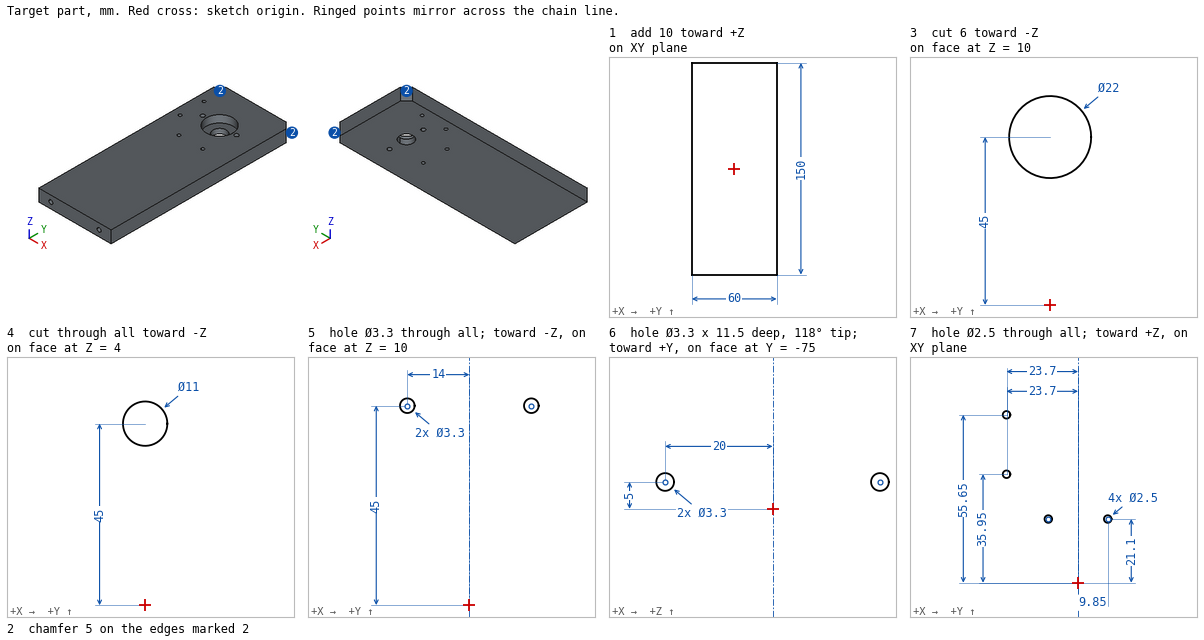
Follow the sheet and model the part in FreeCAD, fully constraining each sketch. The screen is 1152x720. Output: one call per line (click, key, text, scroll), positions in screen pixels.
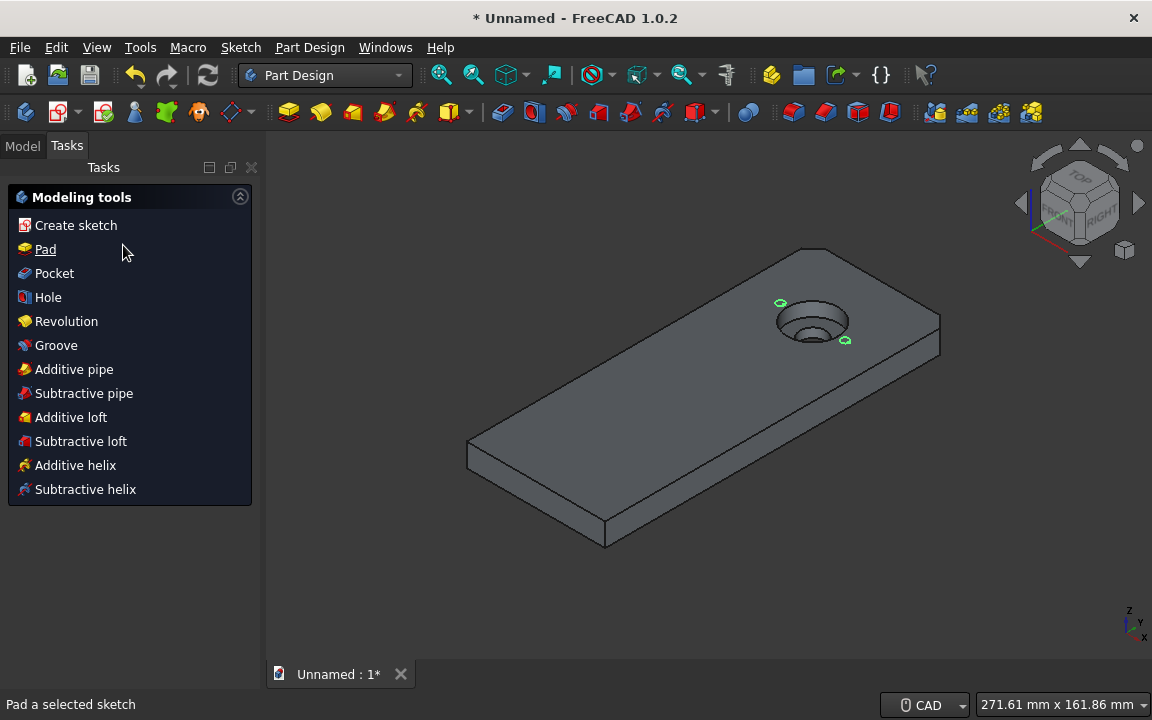
click(536, 112)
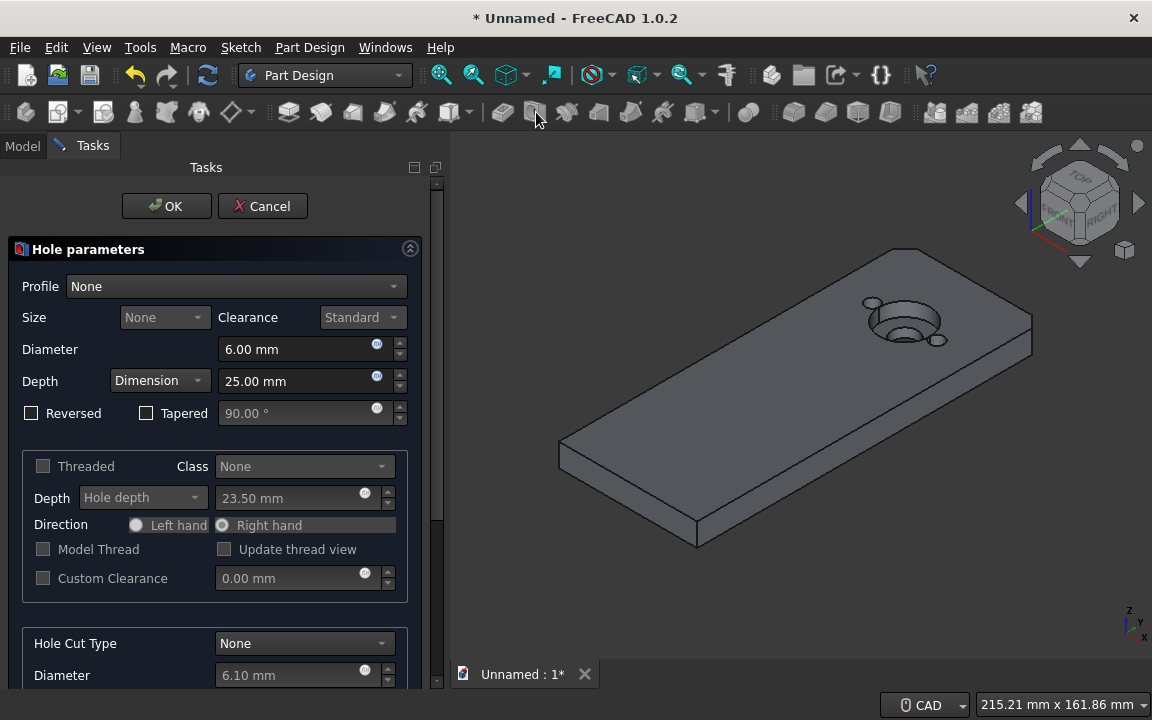
triple_click(305, 349)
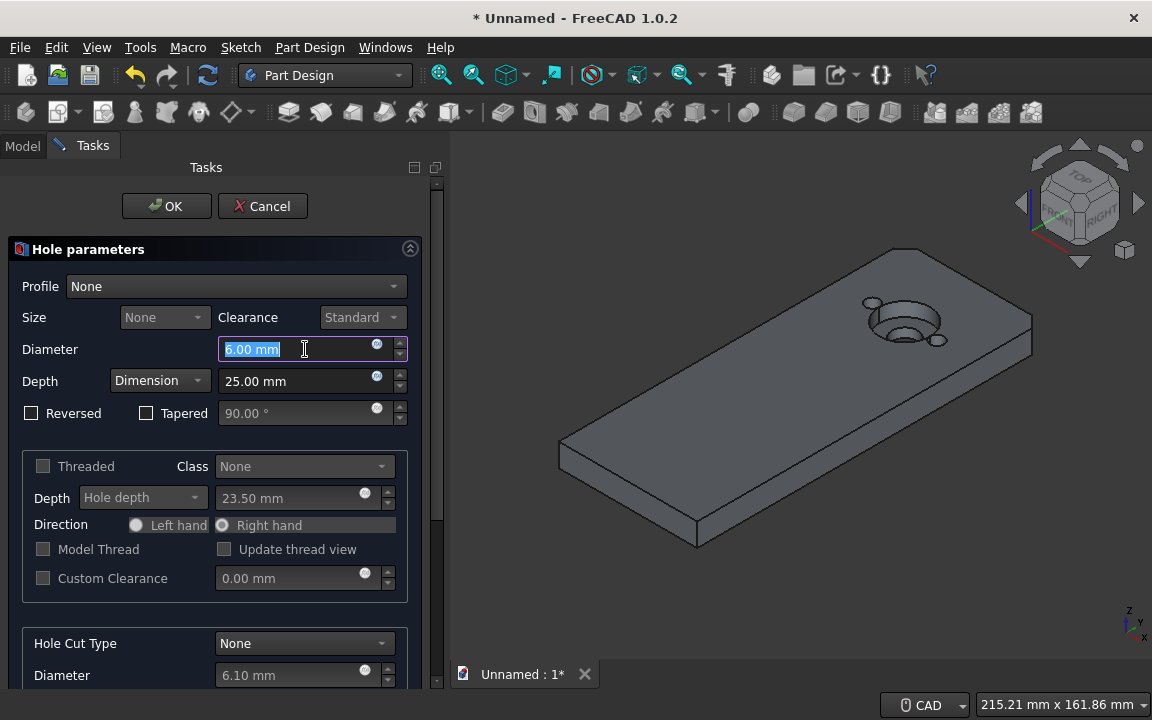
text(3.3)
key(Tab)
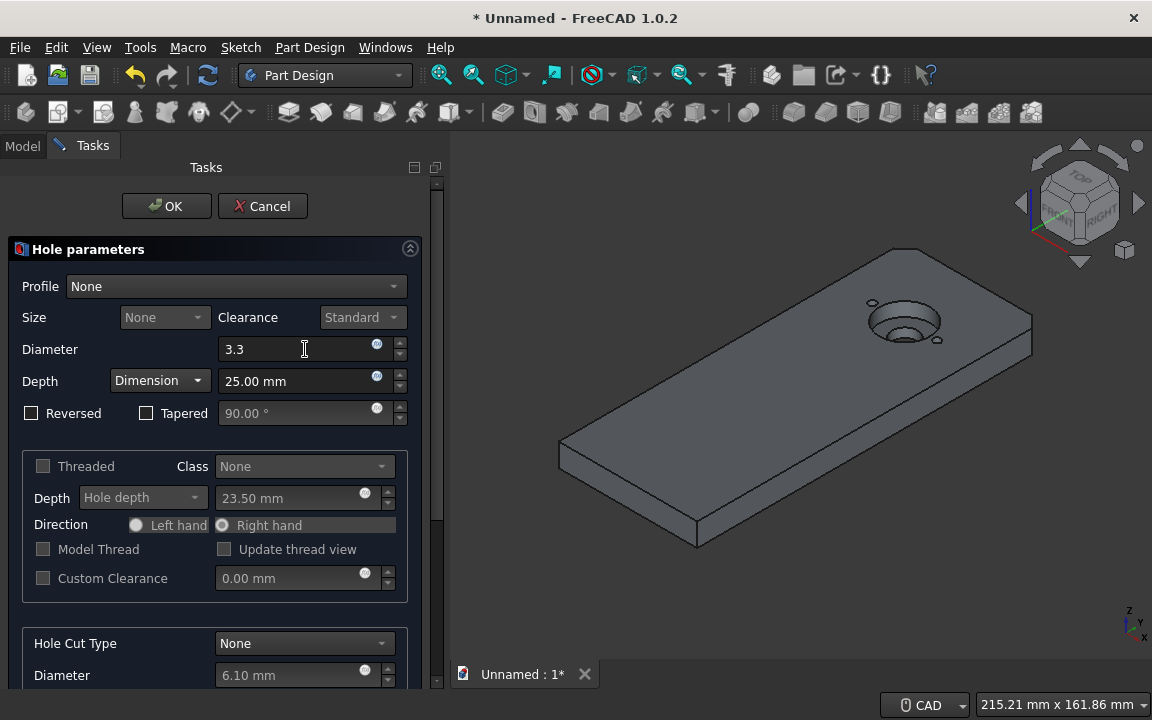
click(161, 380)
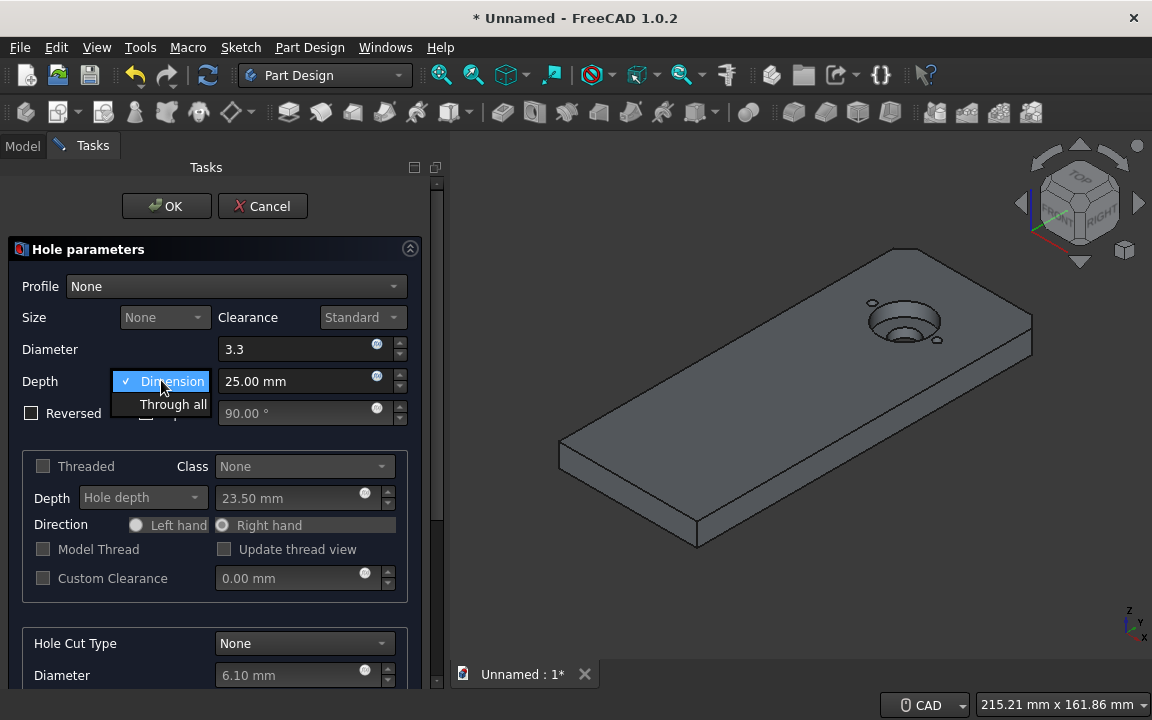
click(160, 404)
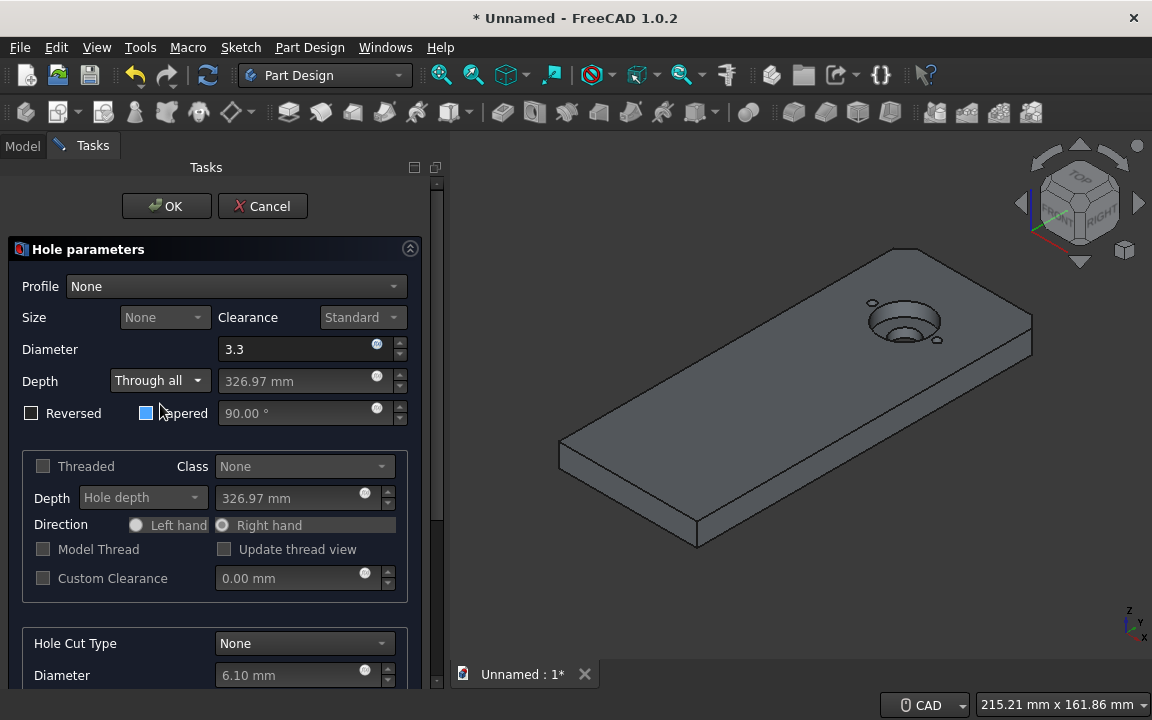
click(167, 206)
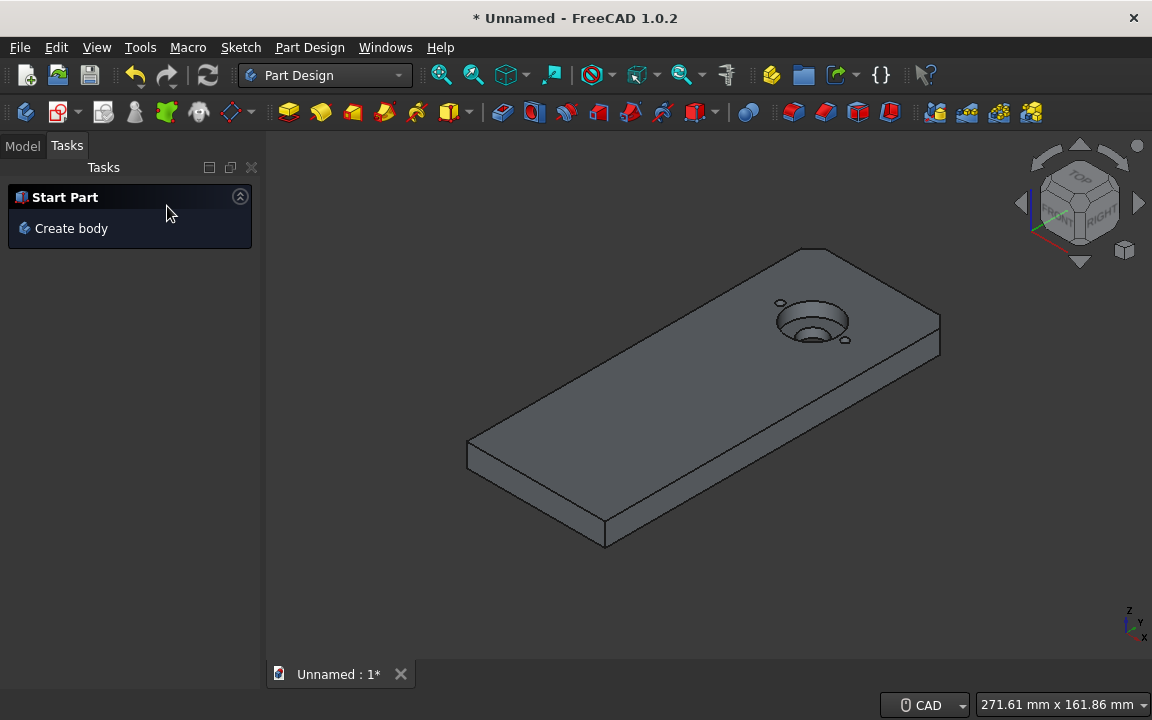
click(576, 517)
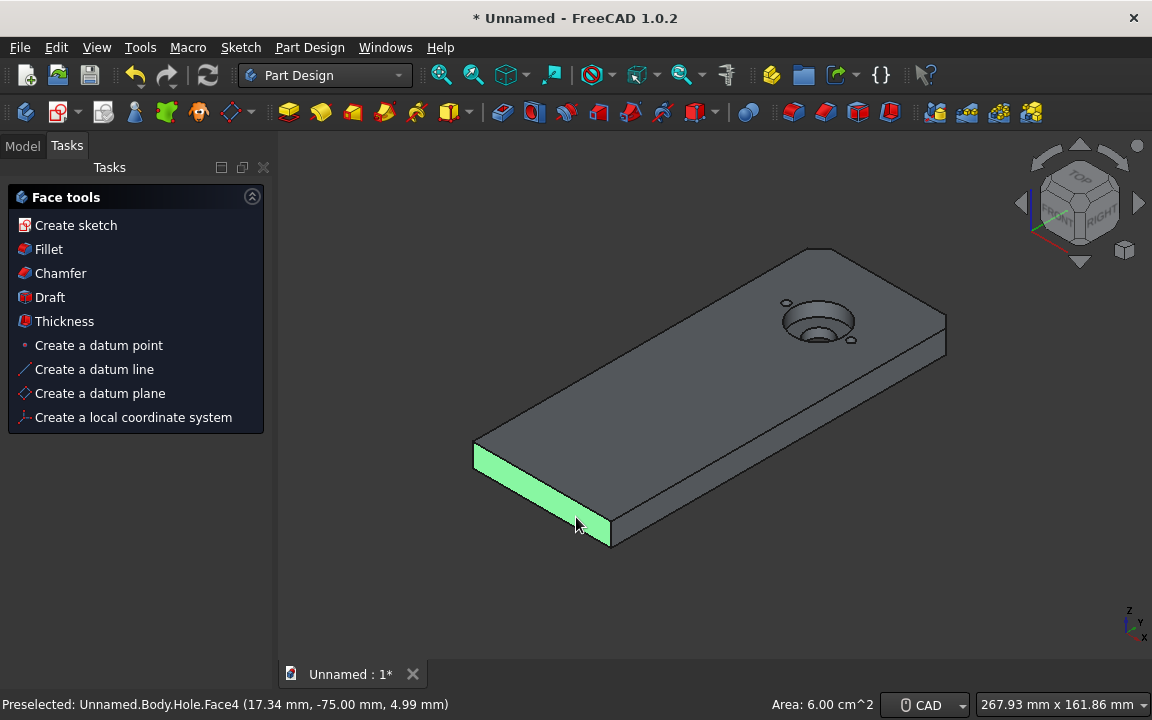
click(58, 112)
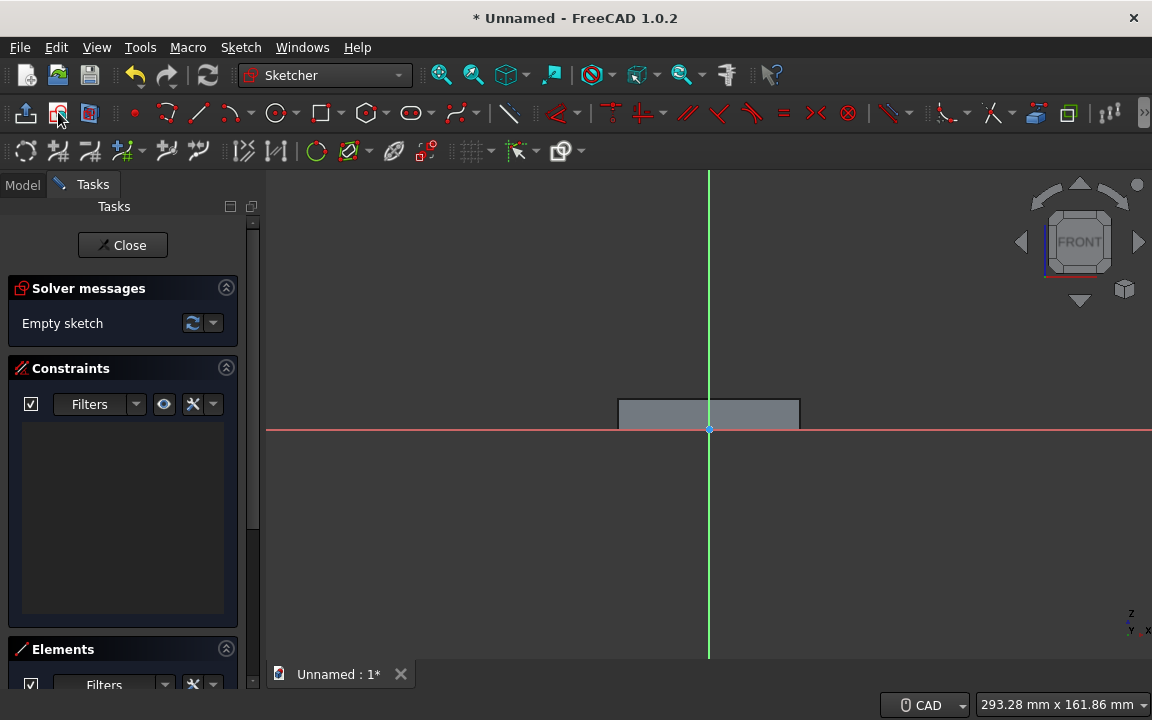
scroll(731, 421, up, 7)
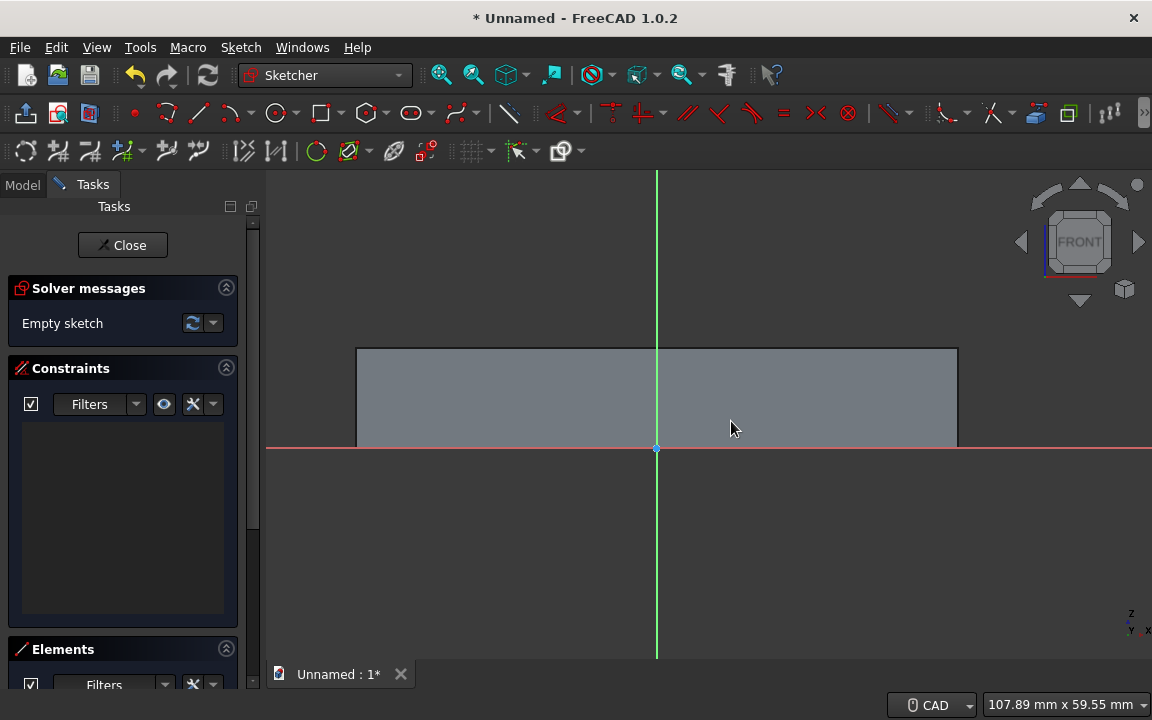
click(276, 114)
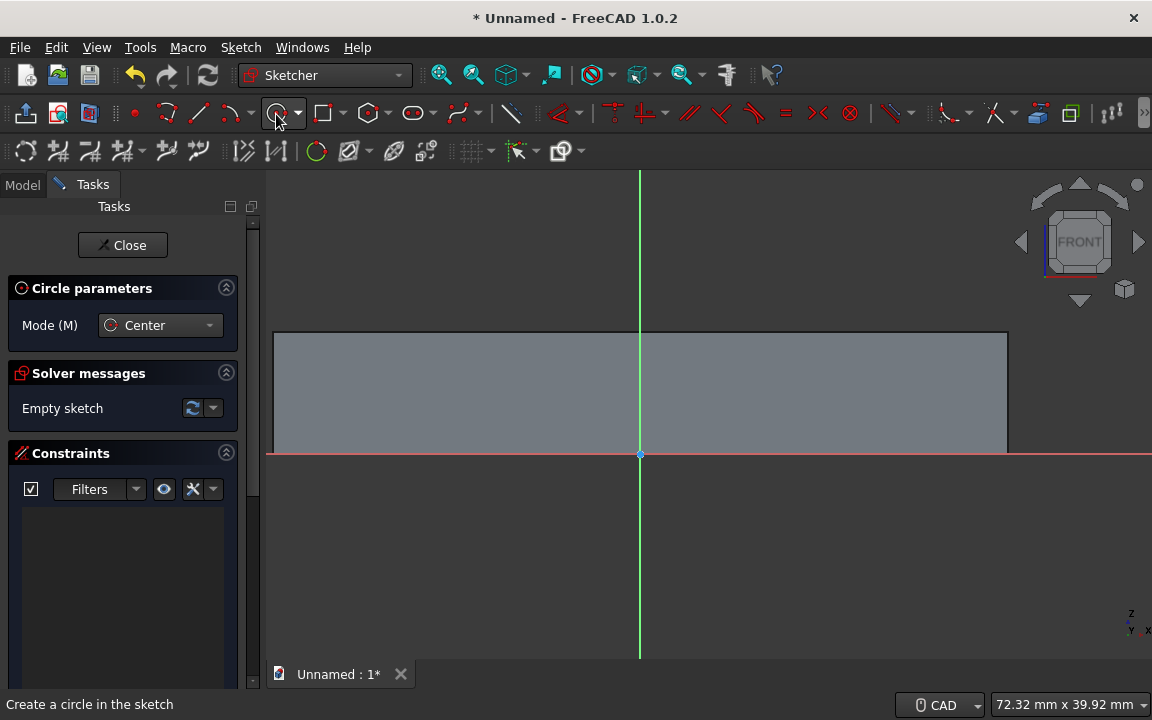
click(395, 393)
click(409, 379)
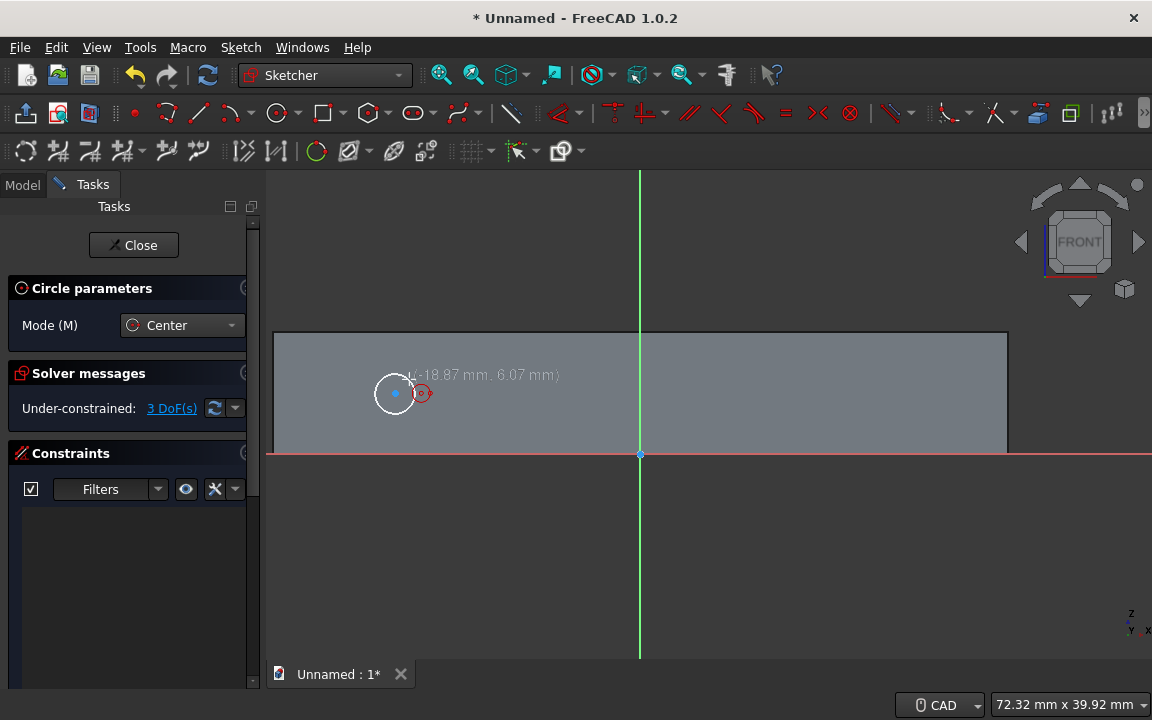
click(885, 393)
click(899, 379)
key(Escape)